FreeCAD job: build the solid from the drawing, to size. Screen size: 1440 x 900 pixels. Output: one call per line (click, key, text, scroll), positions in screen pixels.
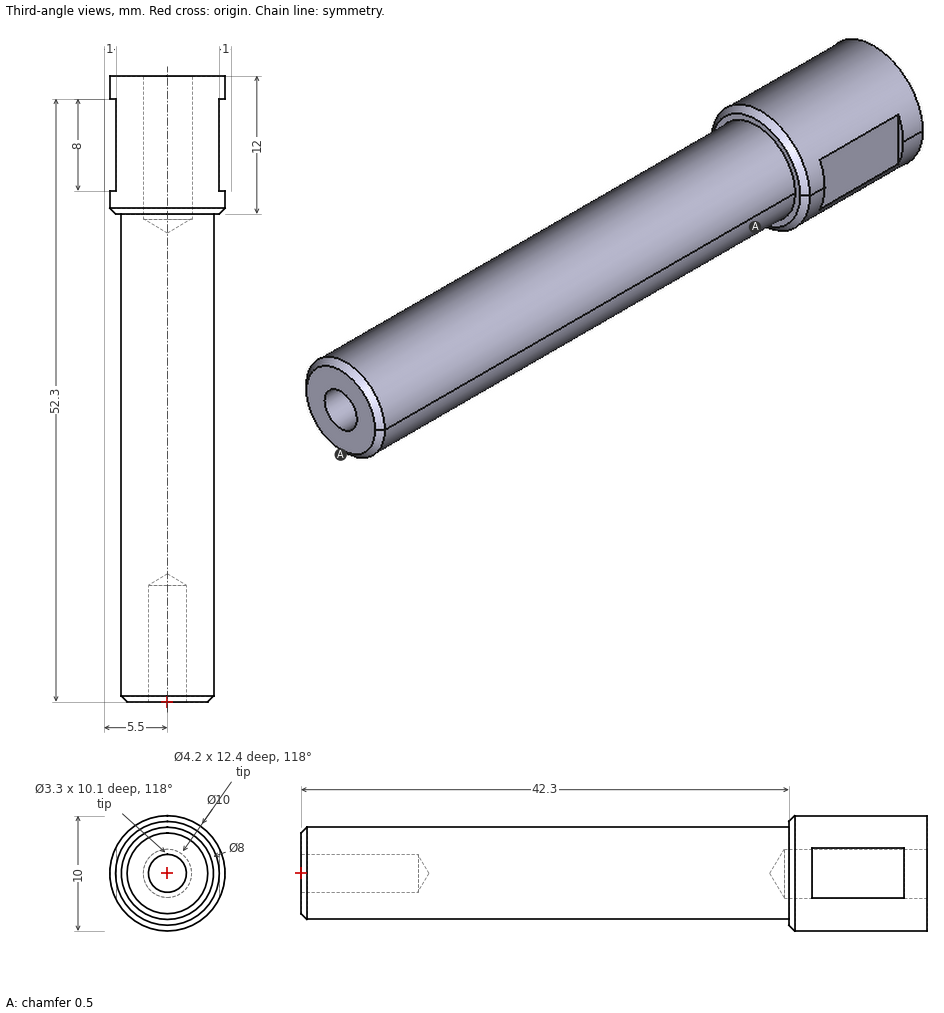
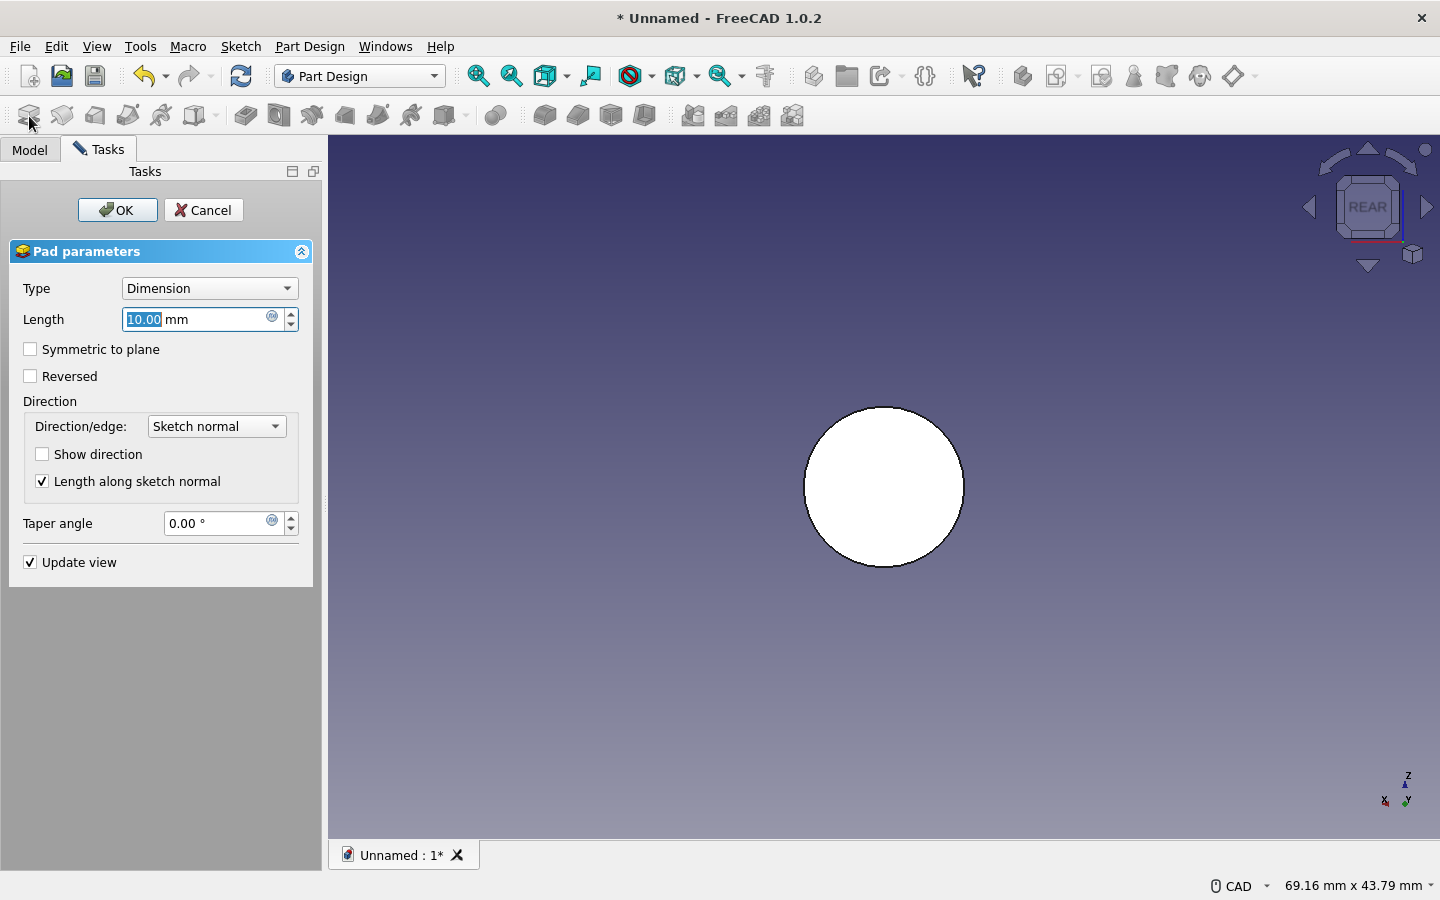
text(12)
key(Tab)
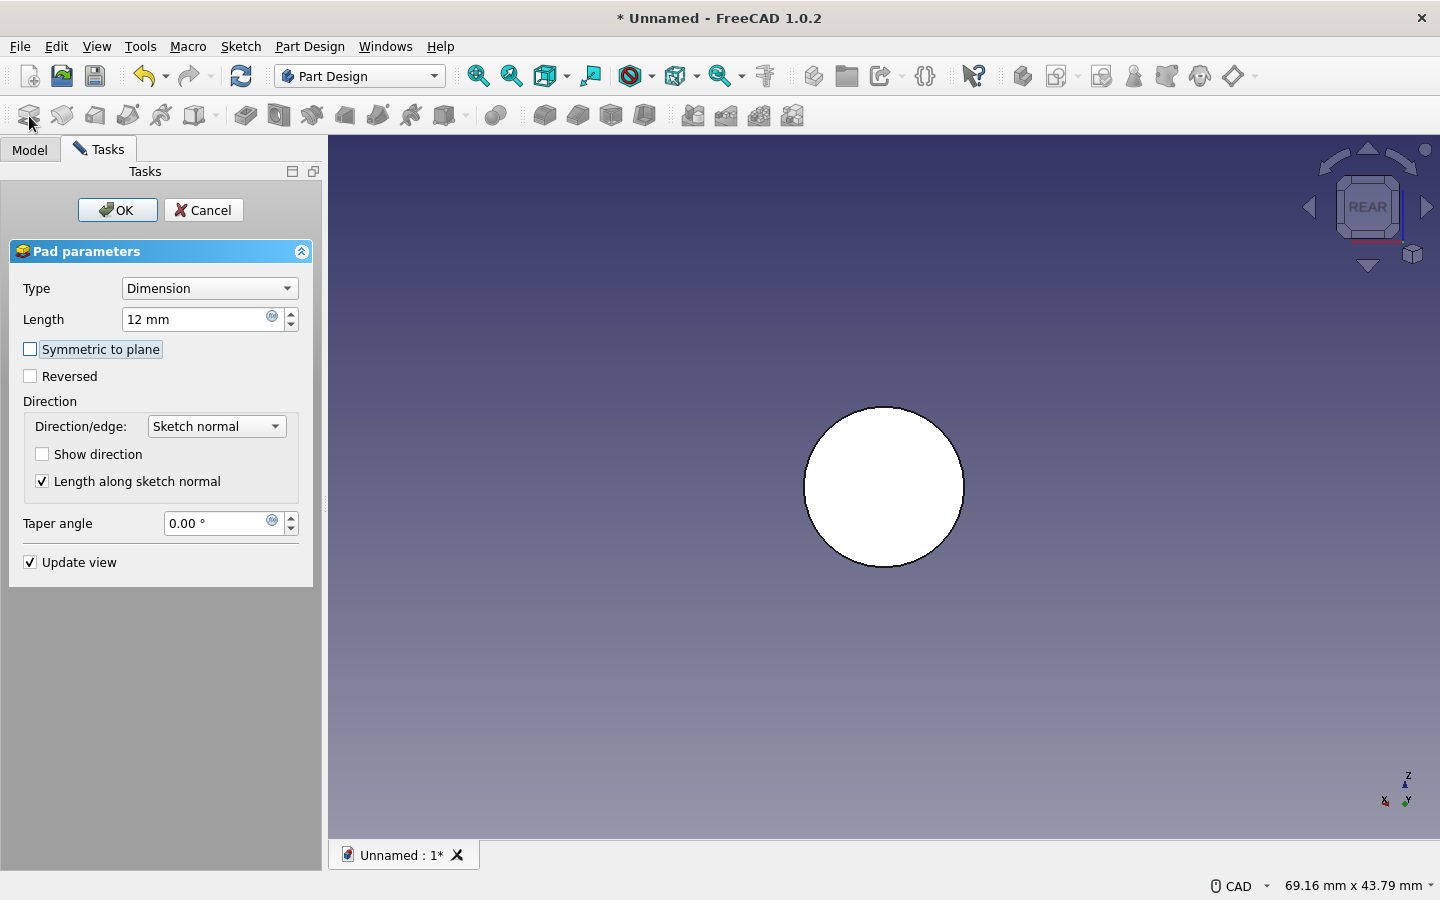
click(118, 210)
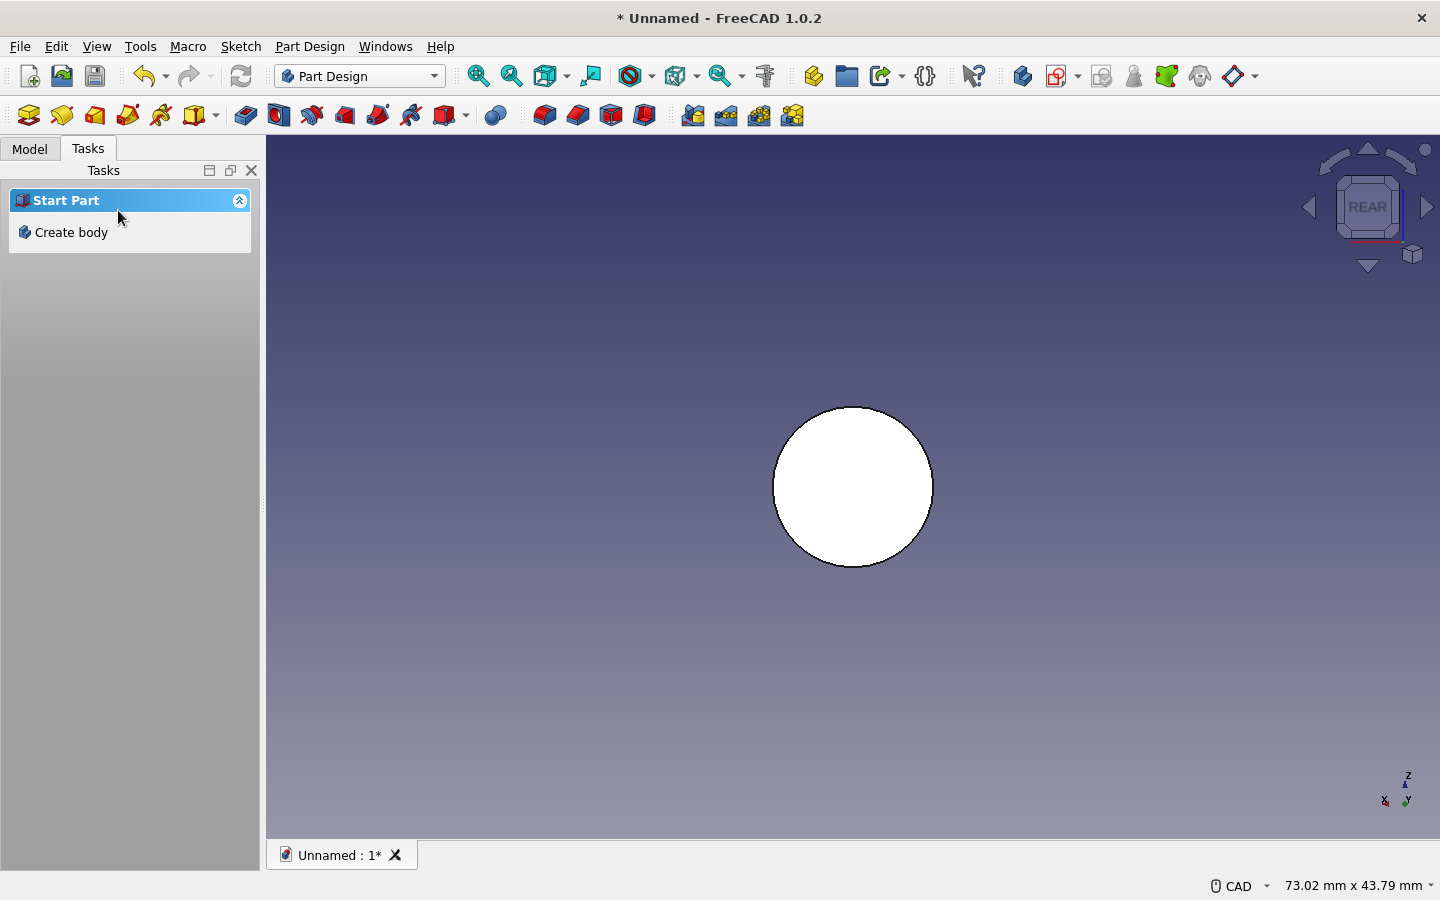
key(v)
key(f)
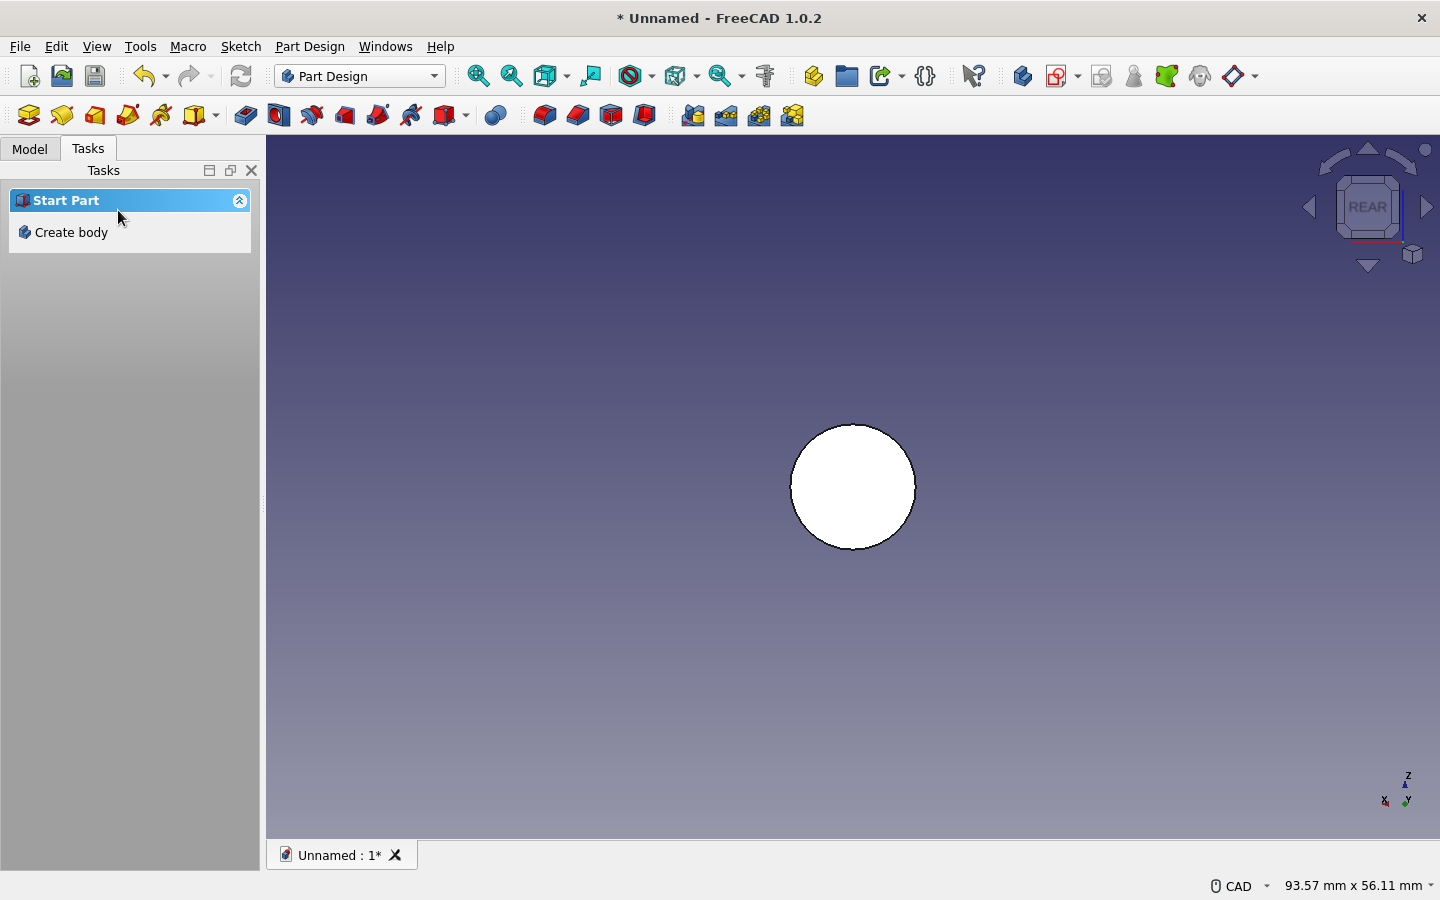
click(853, 486)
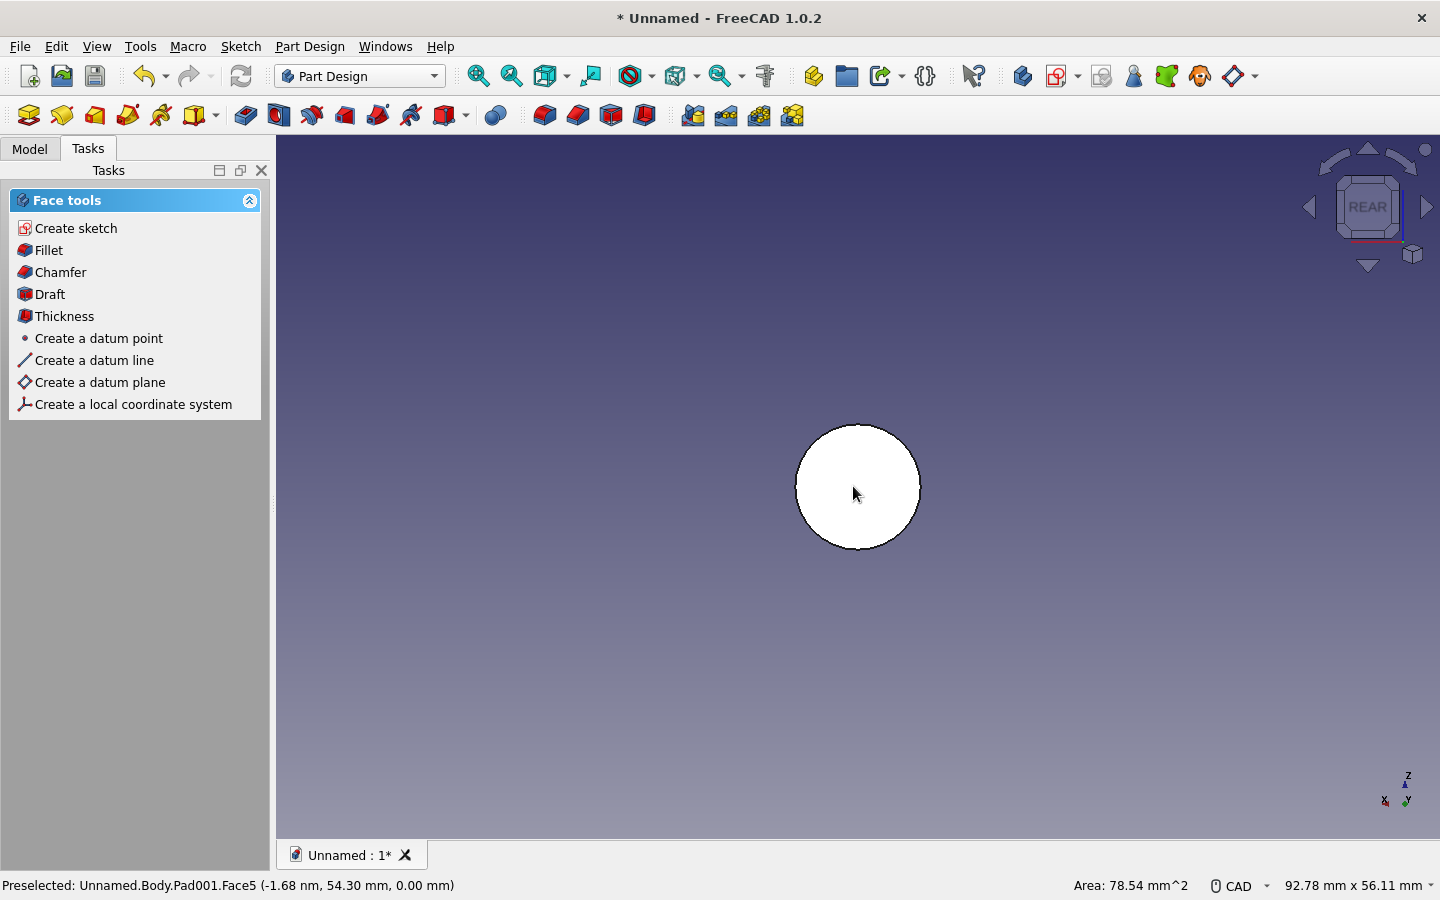
click(1056, 76)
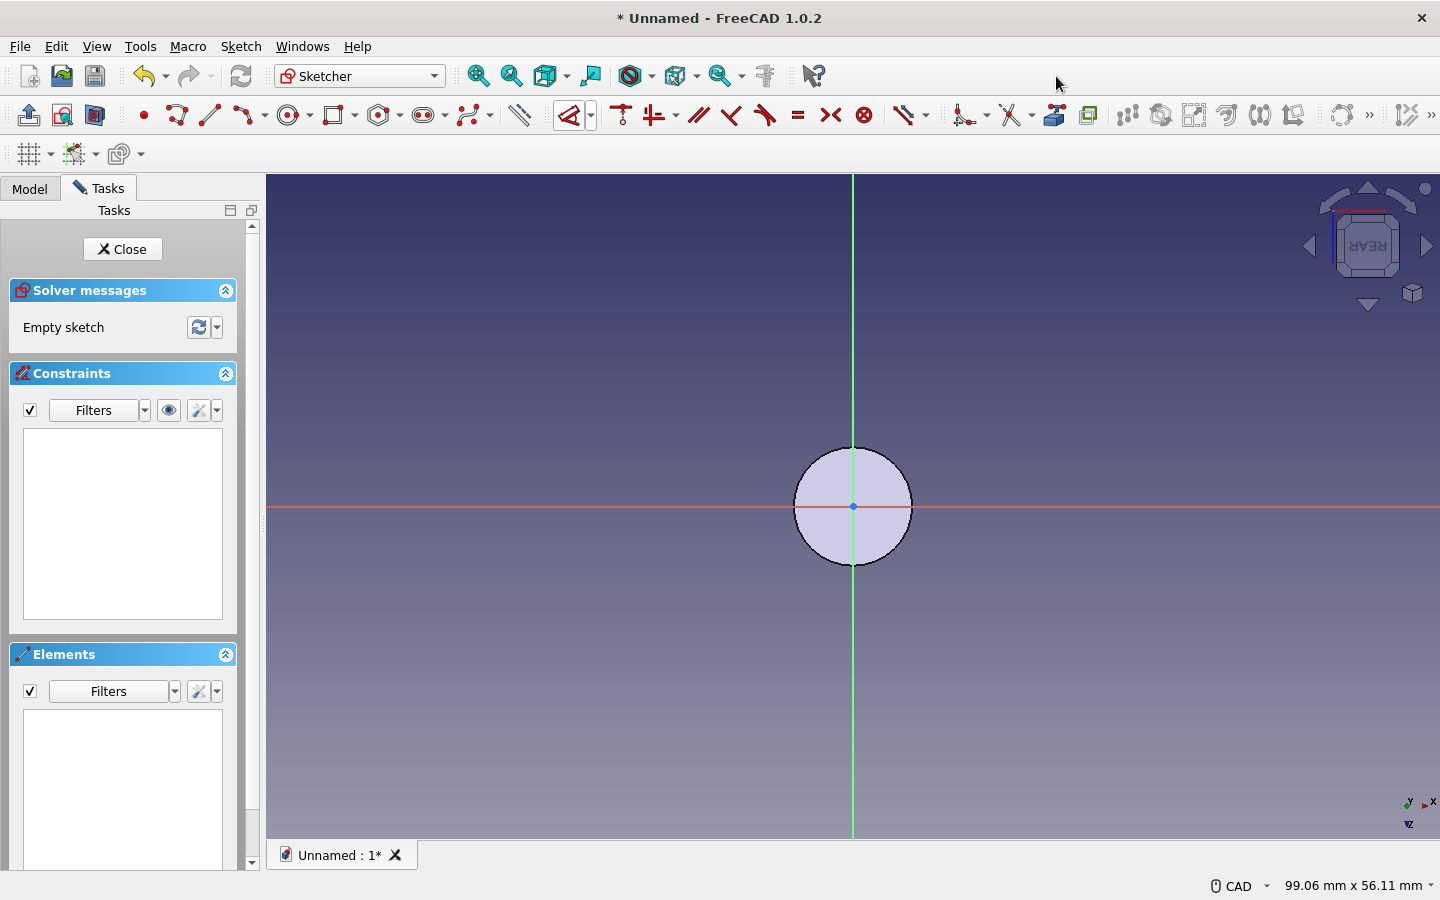
scroll(862, 506, up, 11)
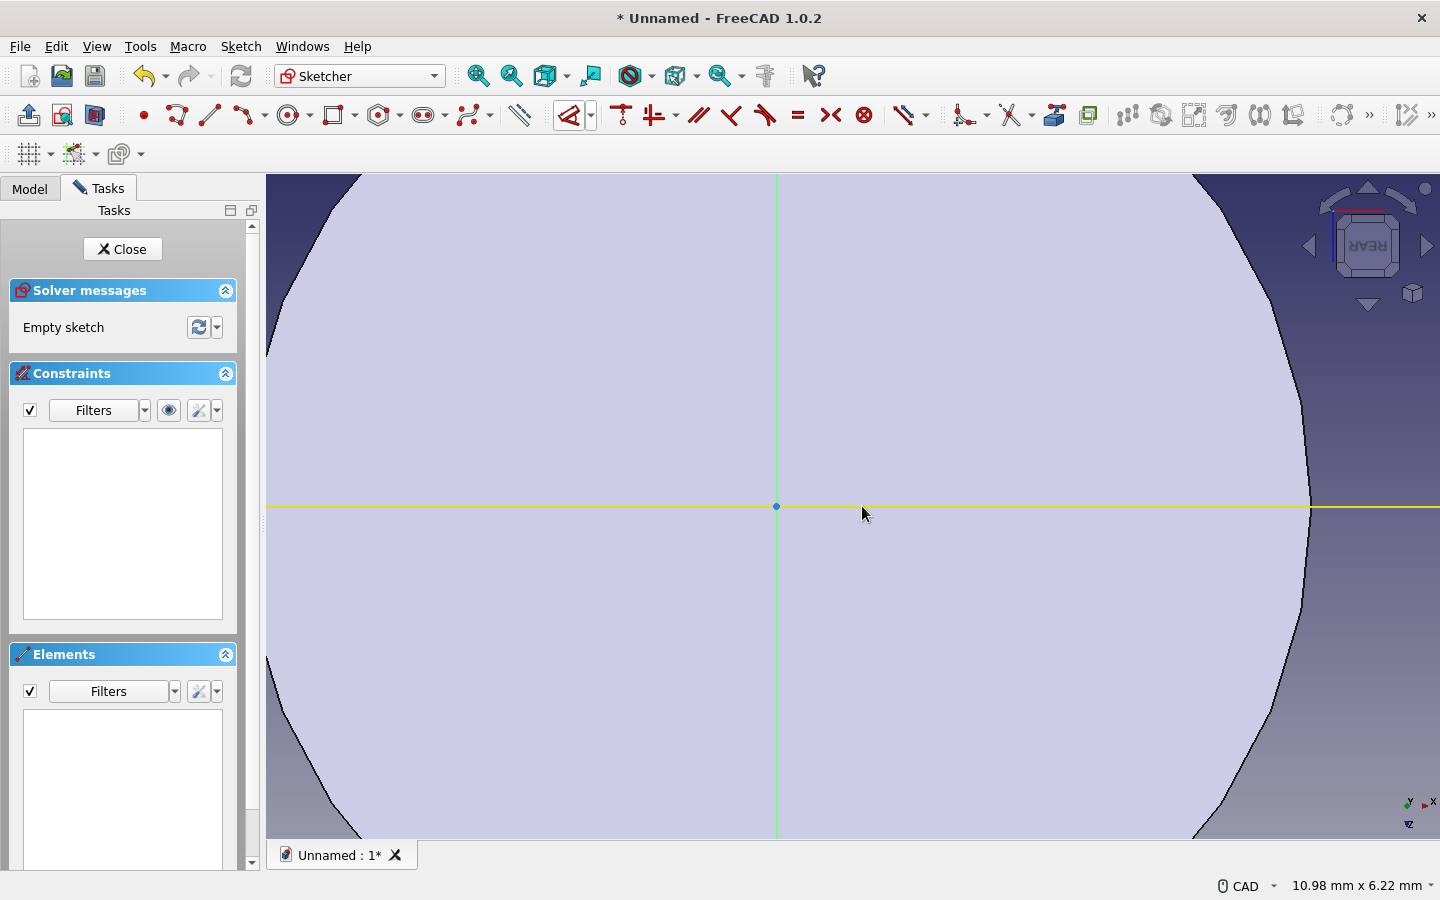
key(g)
key(c)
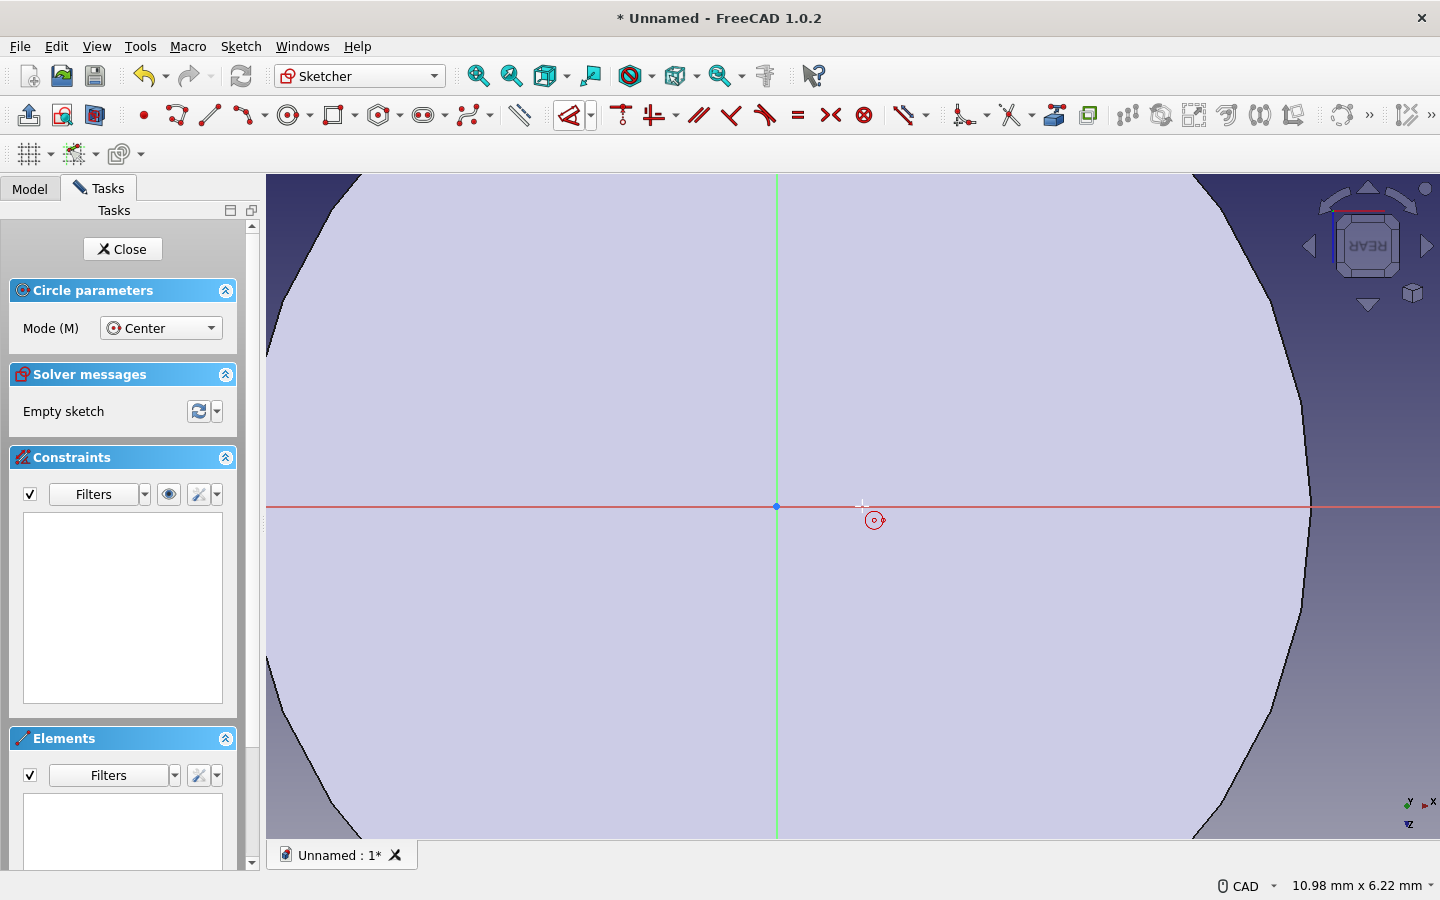
click(777, 506)
move(936, 348)